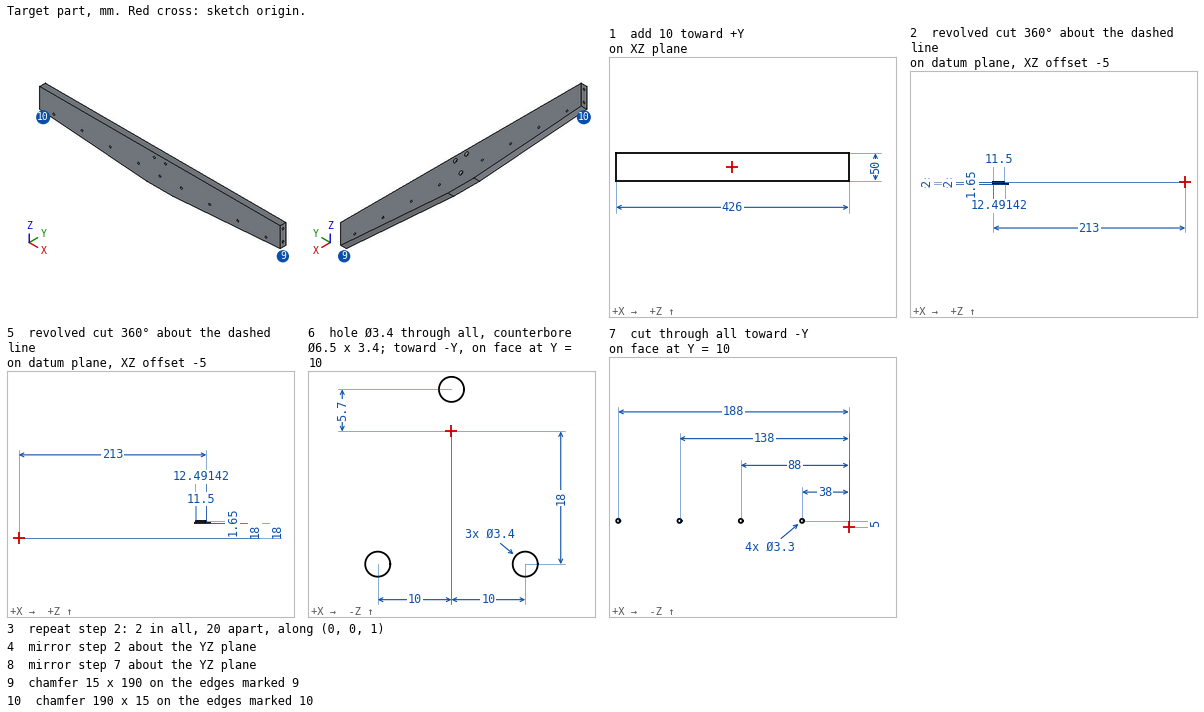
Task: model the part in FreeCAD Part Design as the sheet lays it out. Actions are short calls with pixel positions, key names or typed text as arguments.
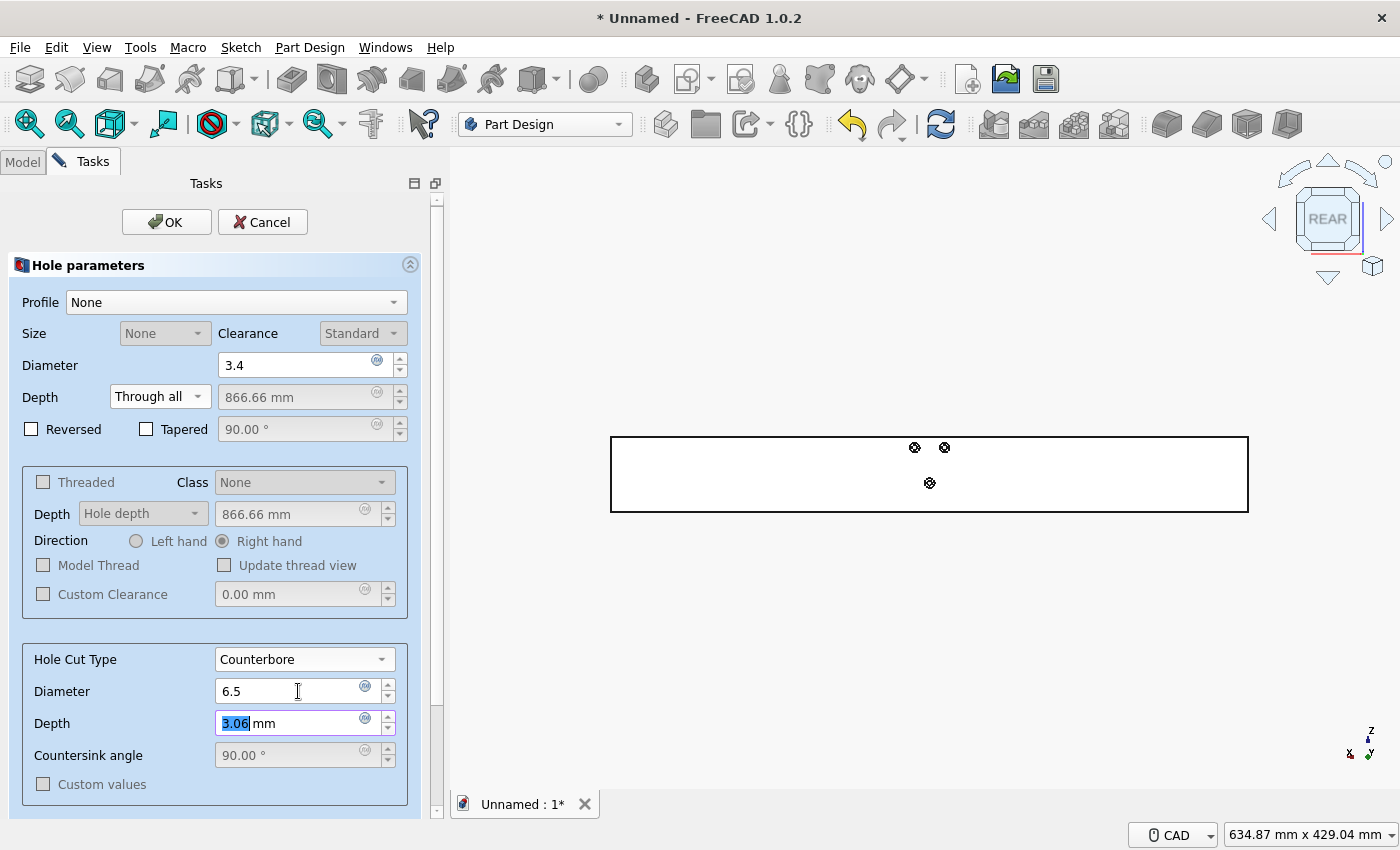
text(3.4)
key(Tab)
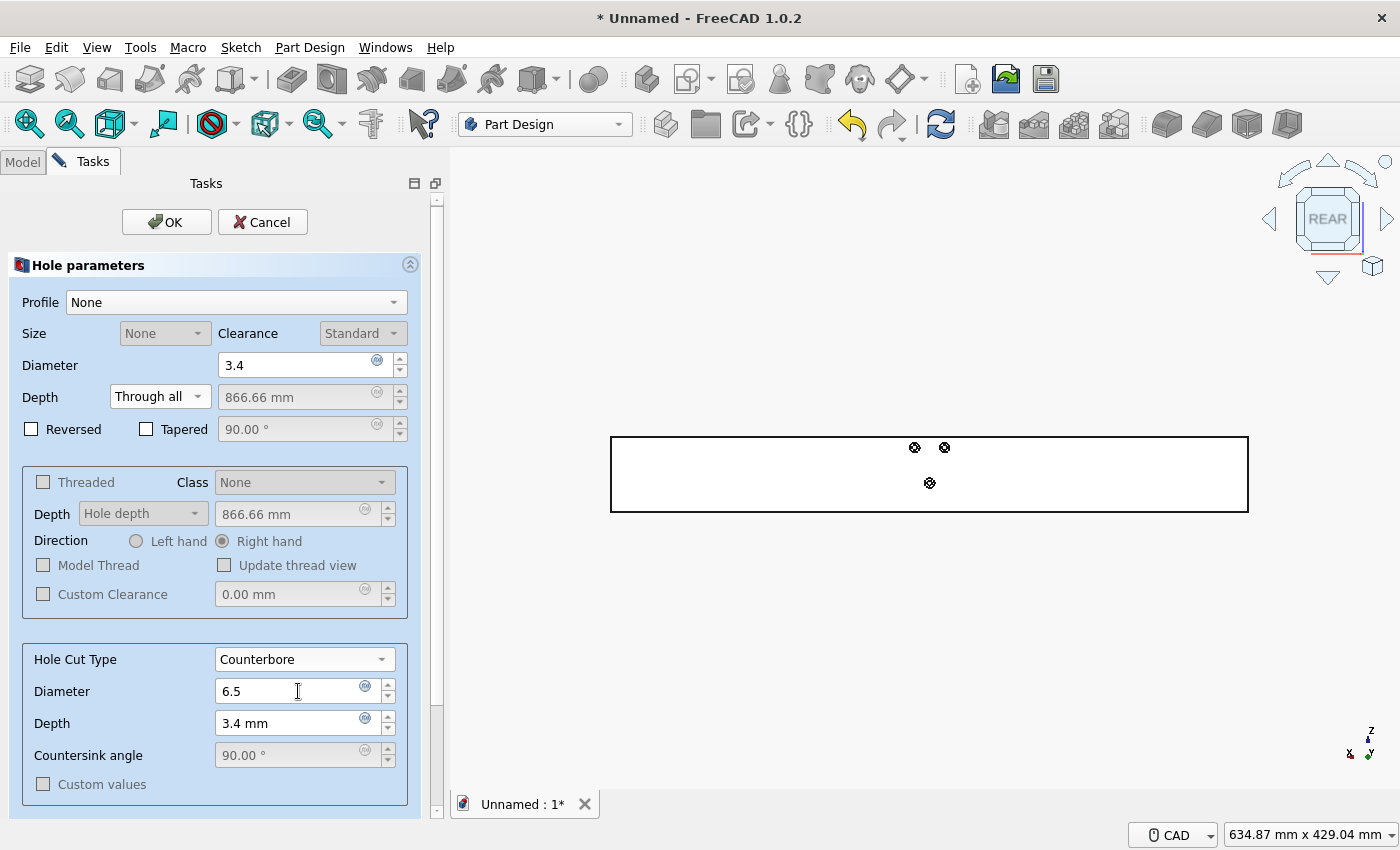
click(167, 222)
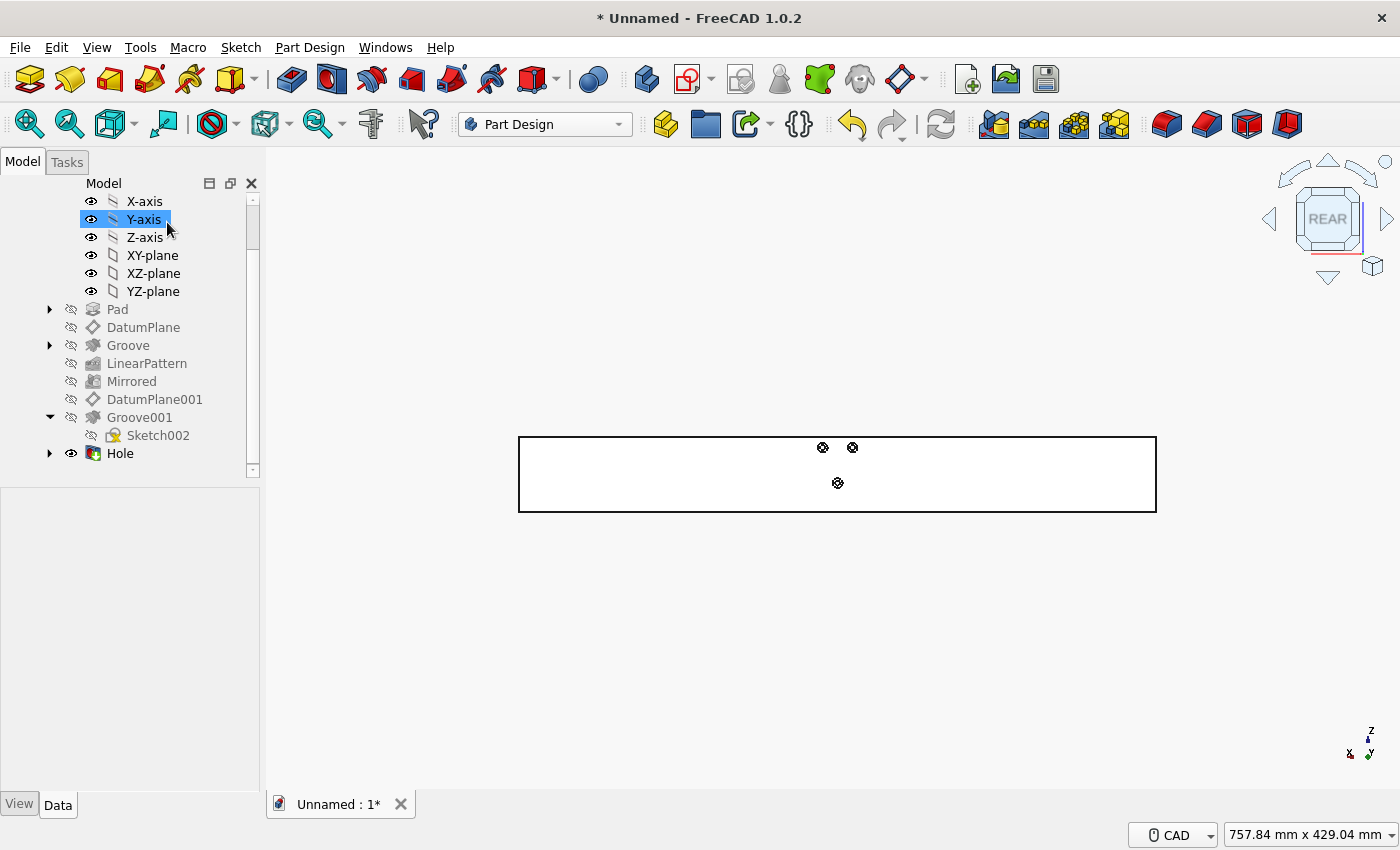
click(564, 474)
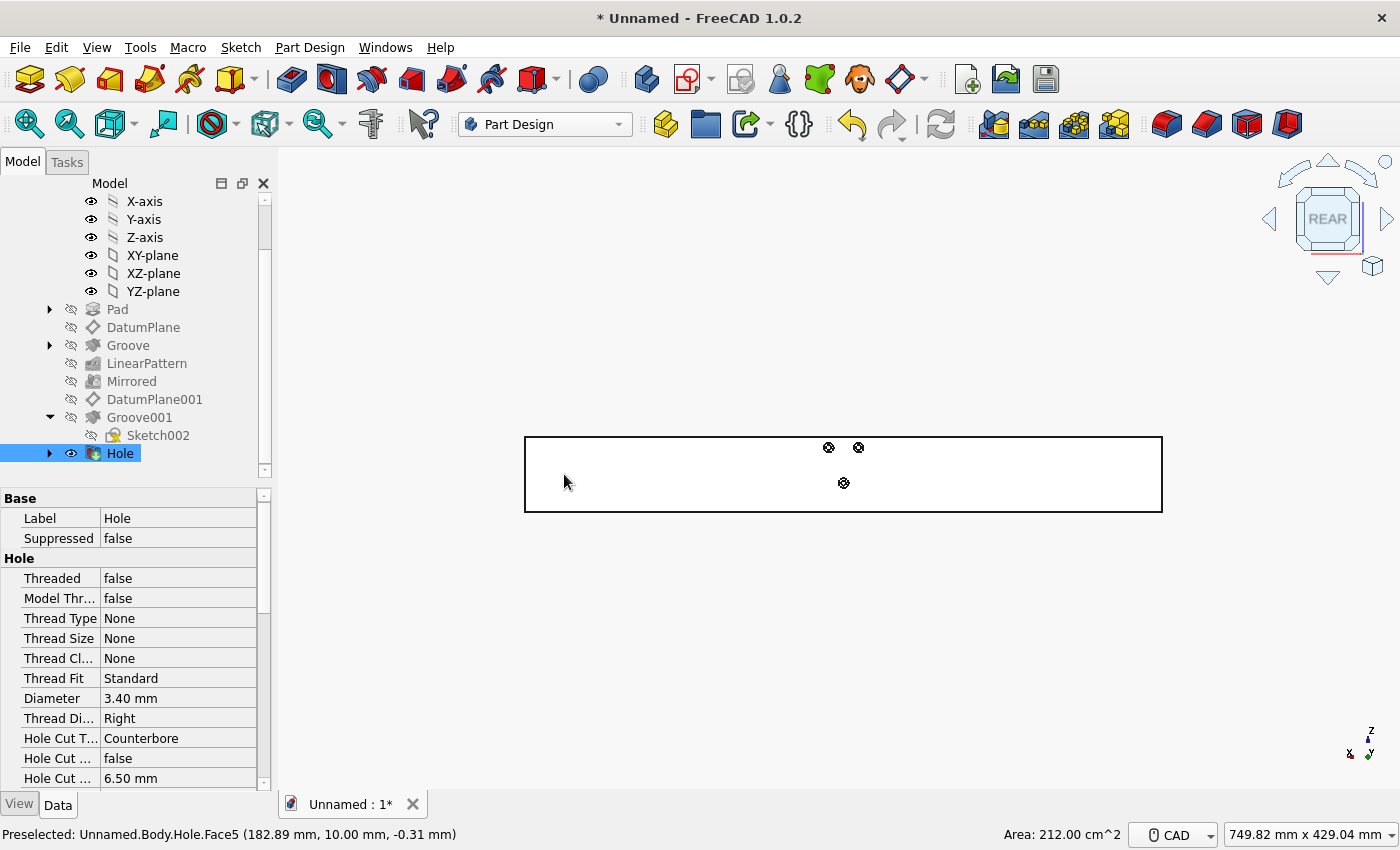
click(688, 80)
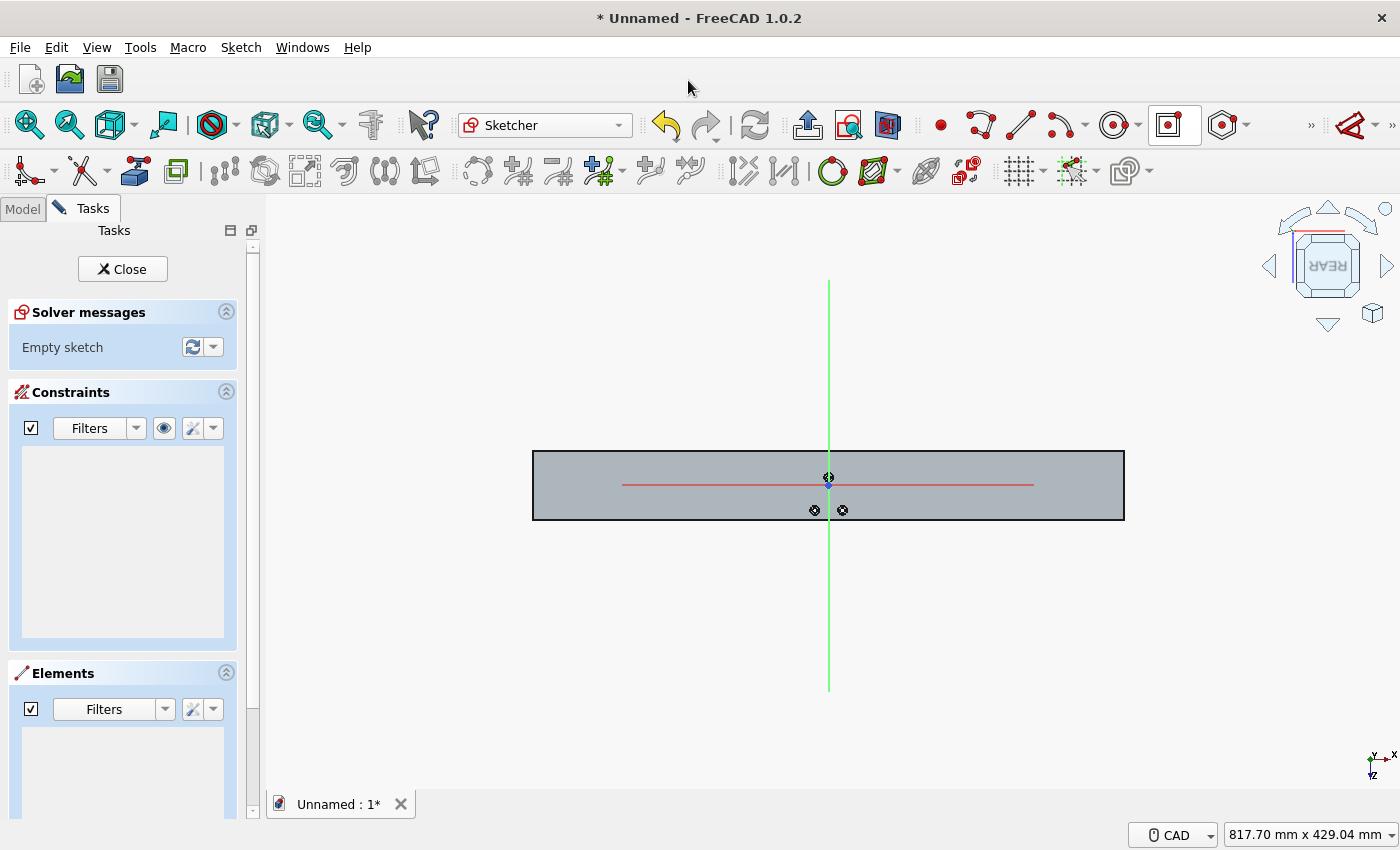
scroll(658, 475, up, 5)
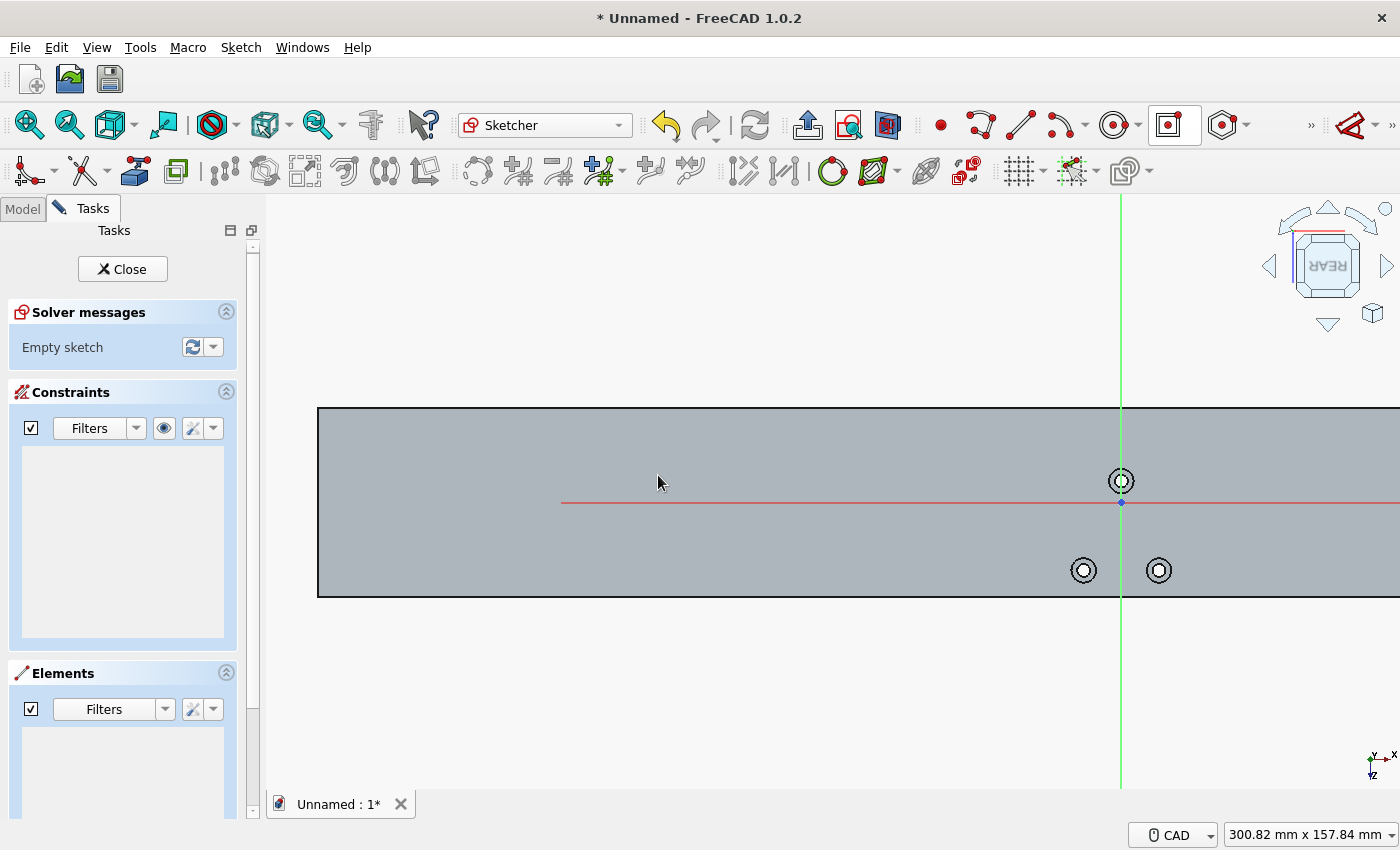
click(1114, 126)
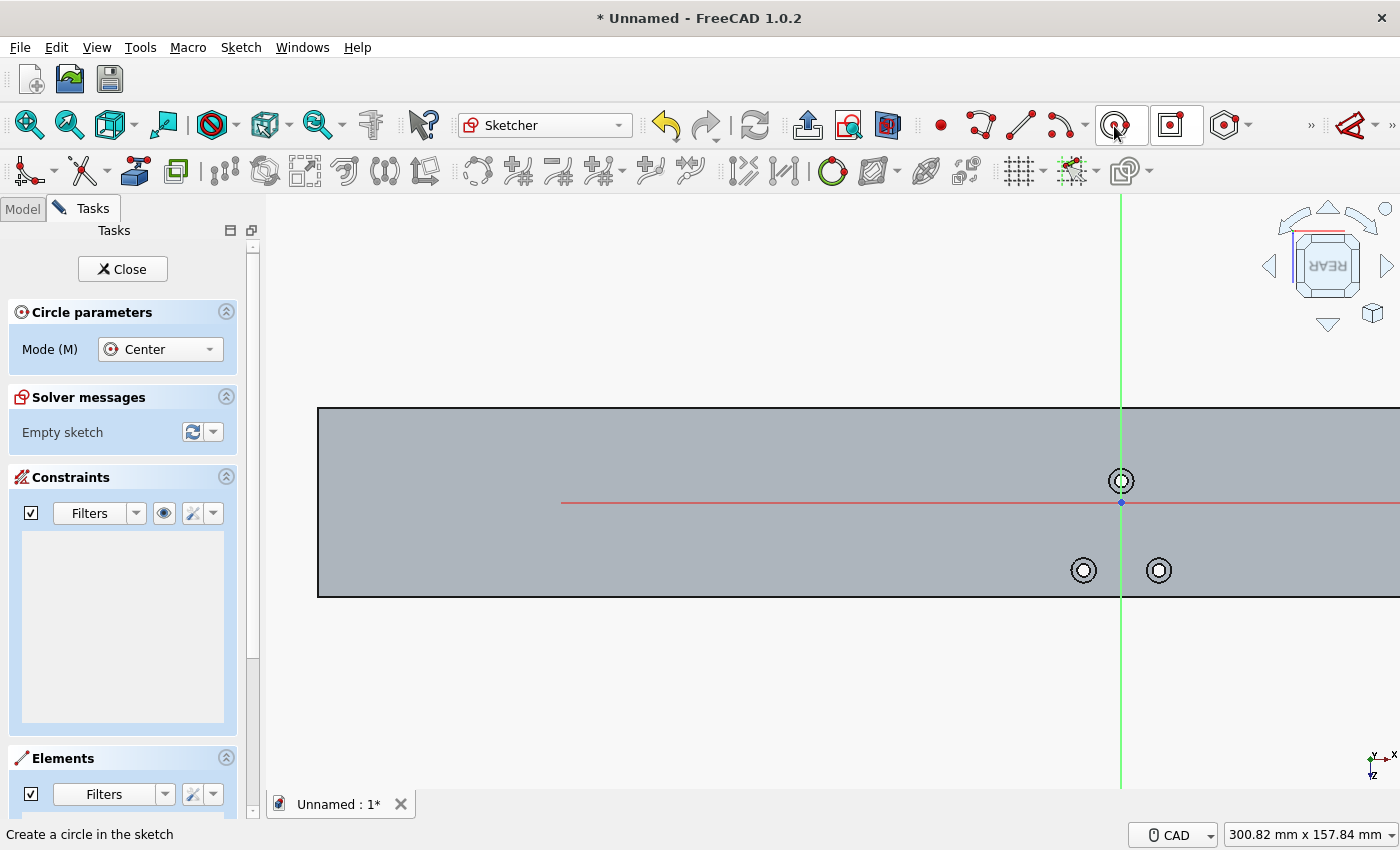
scroll(978, 484, up, 7)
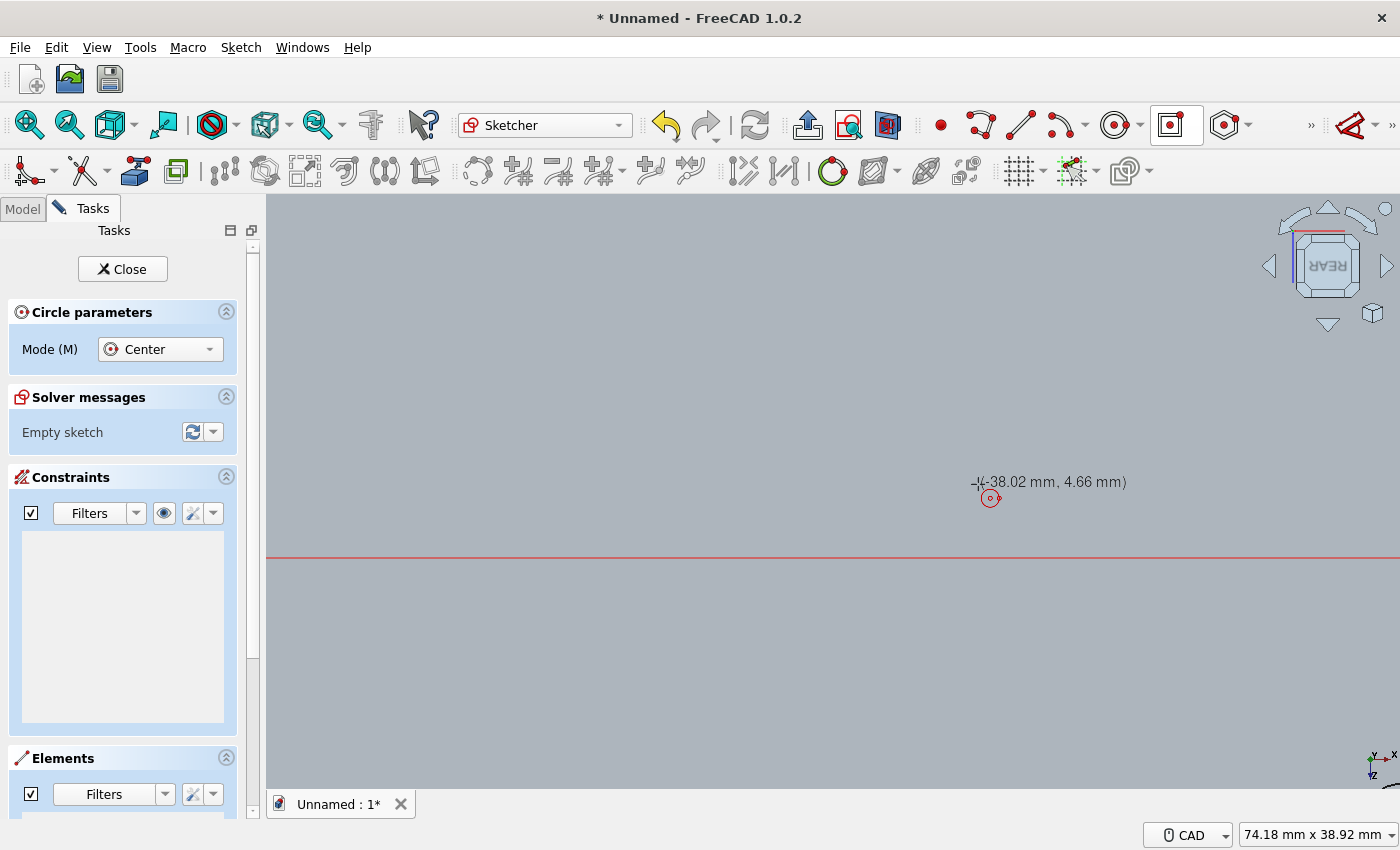
scroll(979, 486, down, 7)